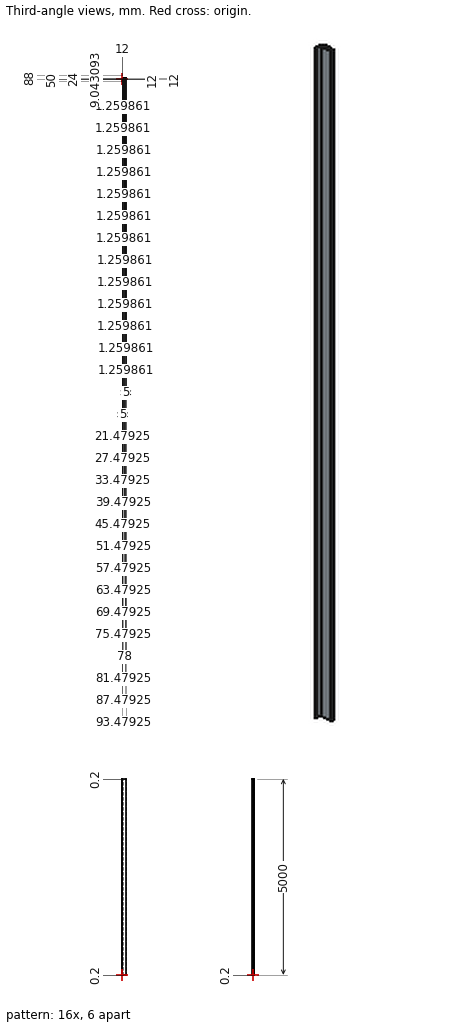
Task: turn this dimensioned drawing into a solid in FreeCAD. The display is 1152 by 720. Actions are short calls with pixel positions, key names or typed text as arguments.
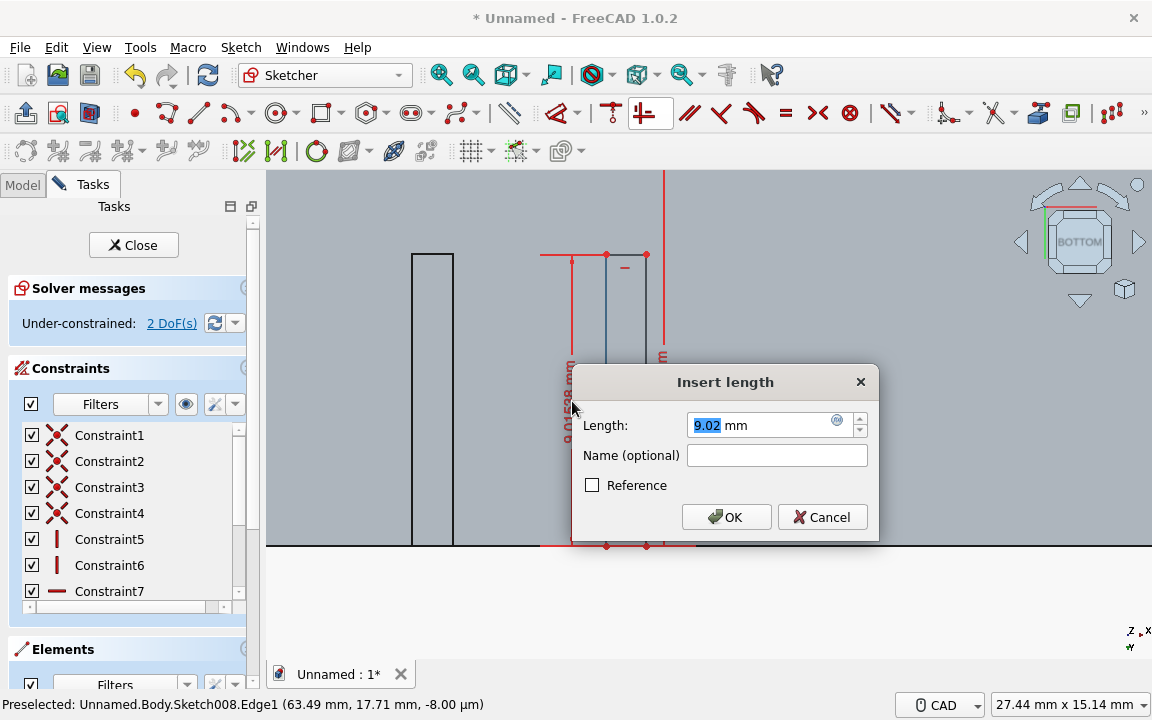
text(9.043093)
key(Return)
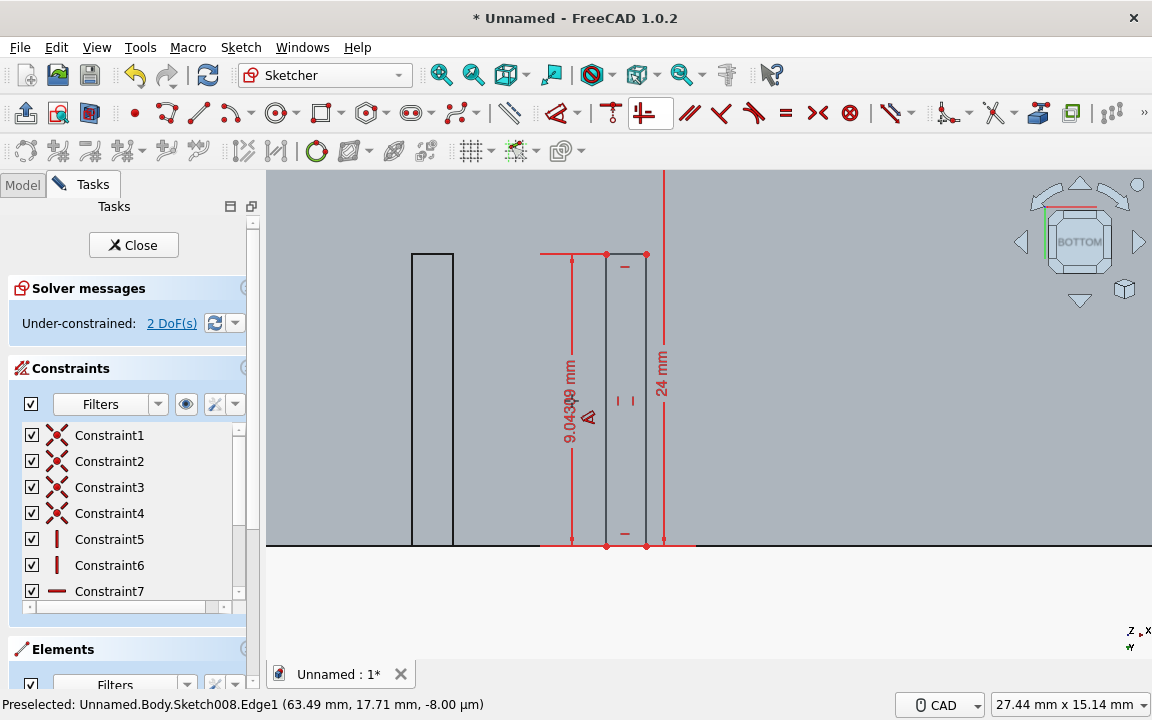
click(618, 546)
click(626, 580)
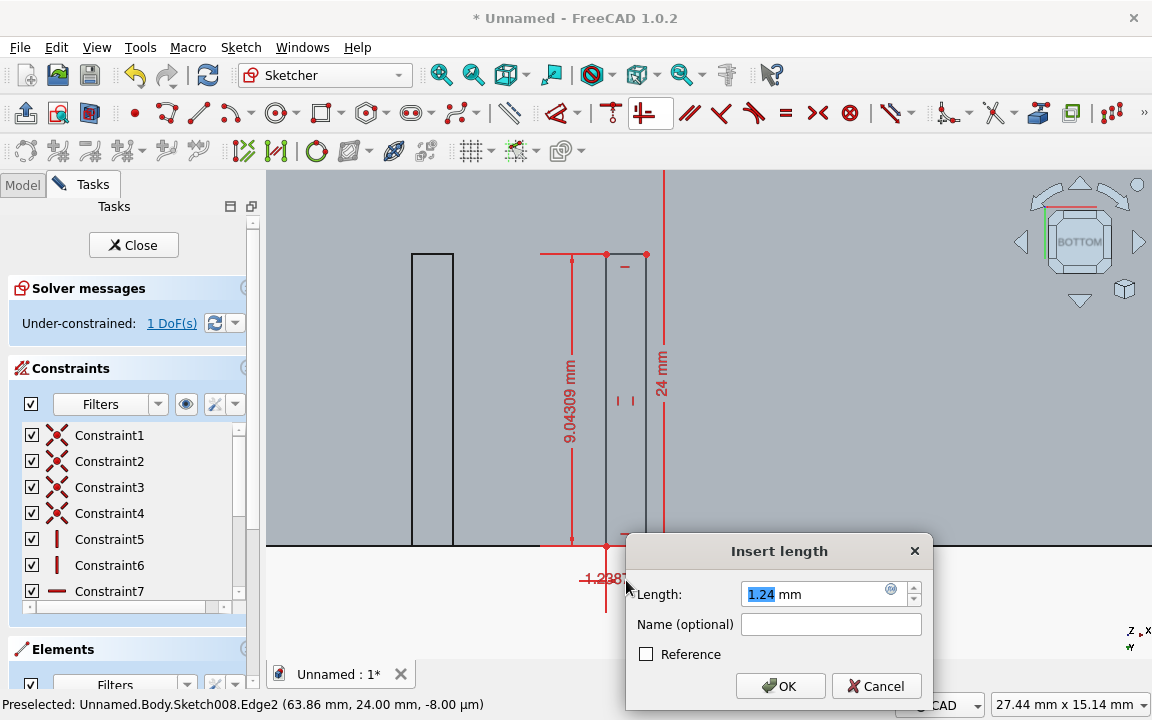
text(1.259861)
key(Return)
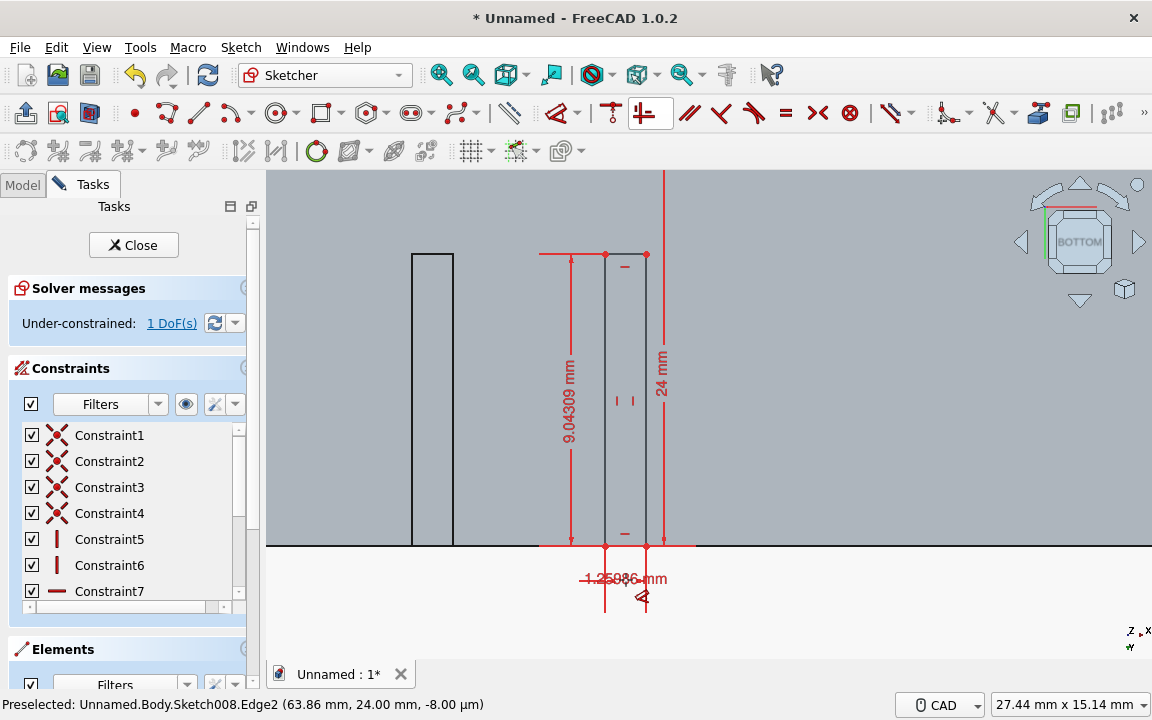
click(605, 254)
click(450, 288)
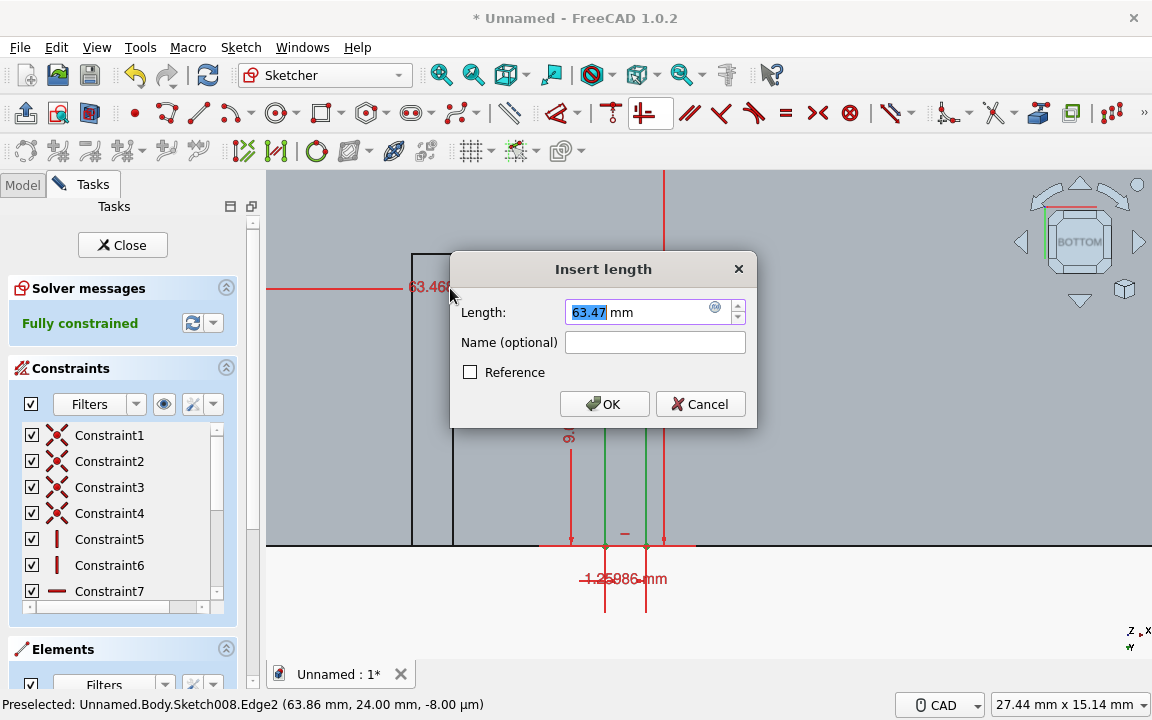
text(63.47925)
key(Return)
key(Escape)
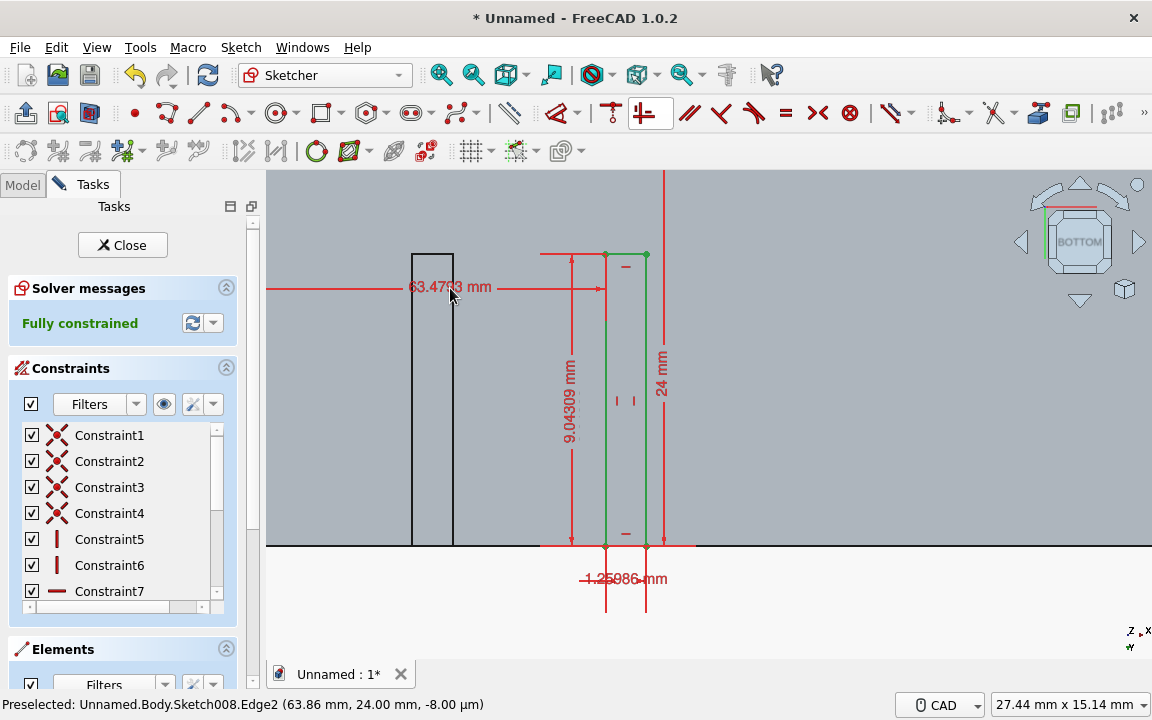
click(123, 245)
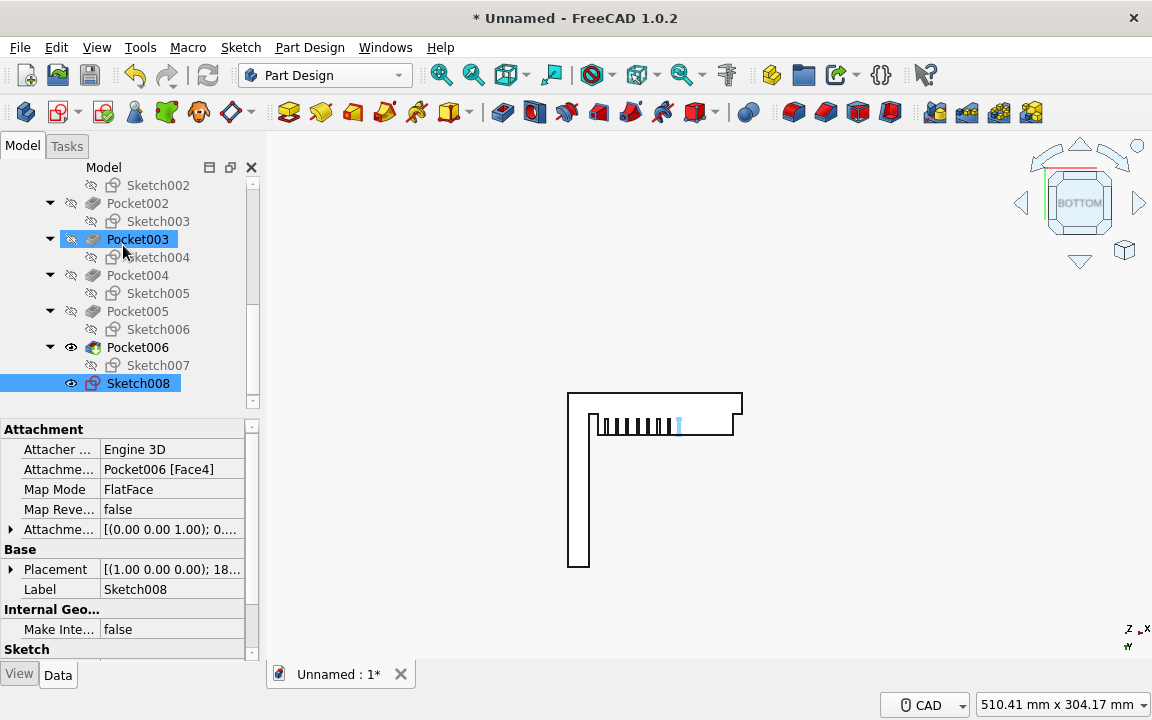
click(504, 112)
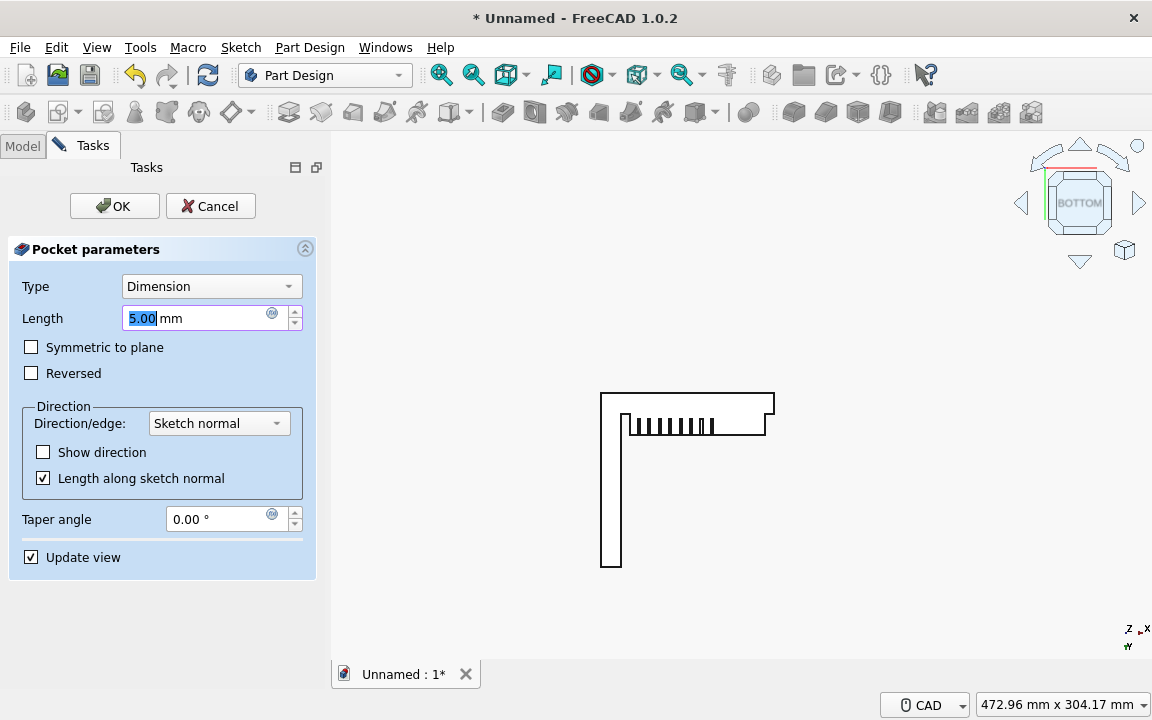
text(0.2)
key(Tab)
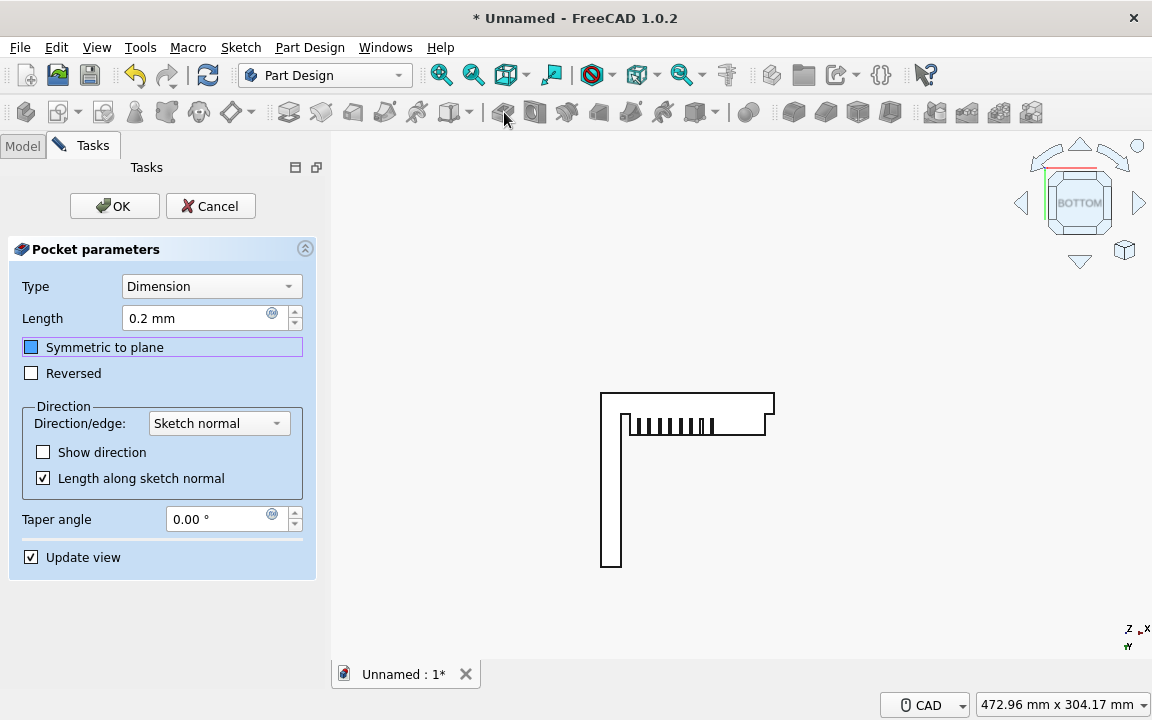
click(115, 206)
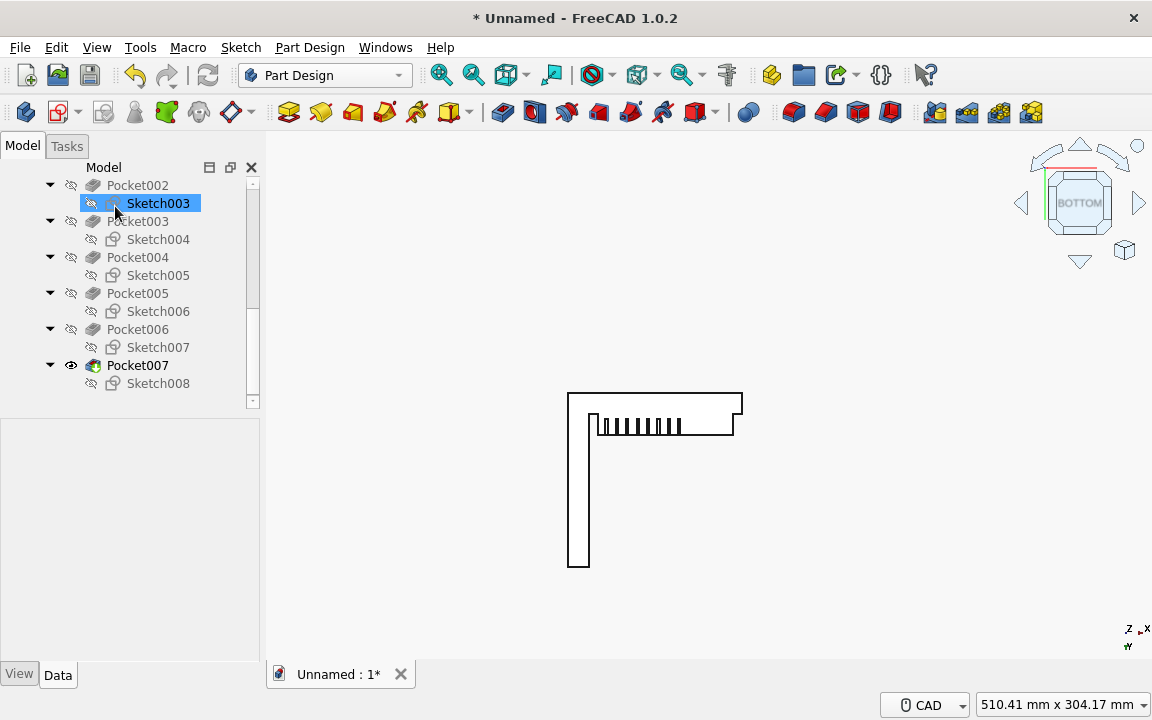
click(442, 76)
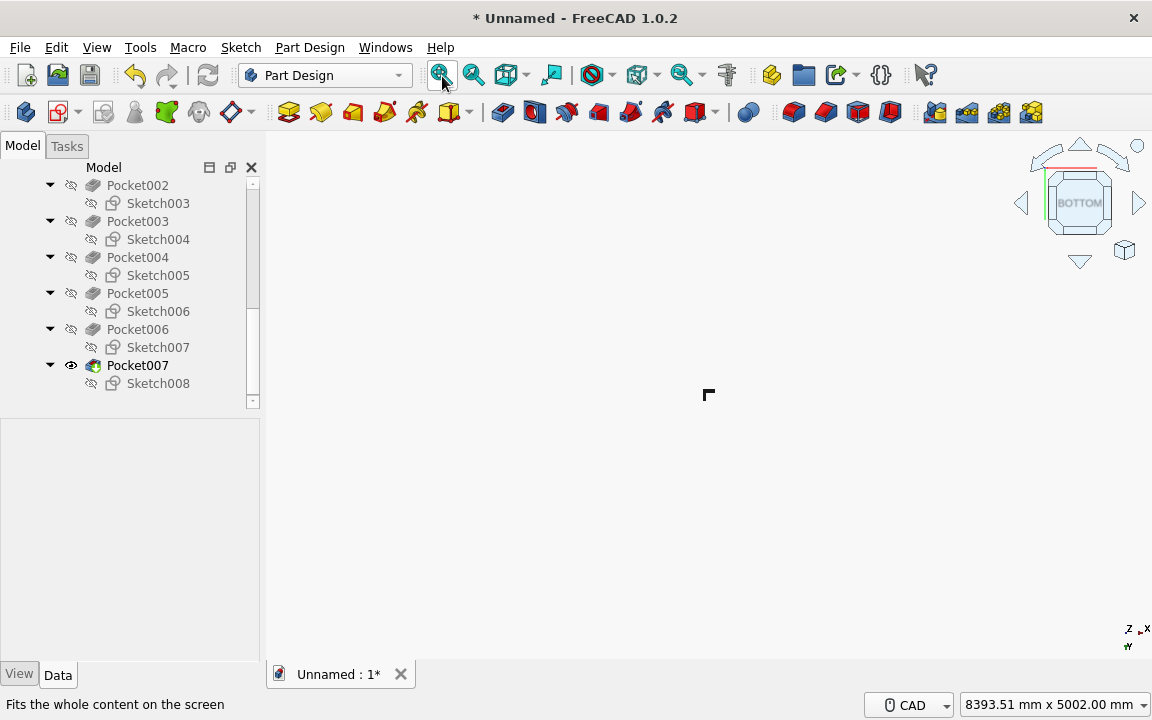
scroll(712, 389, up, 14)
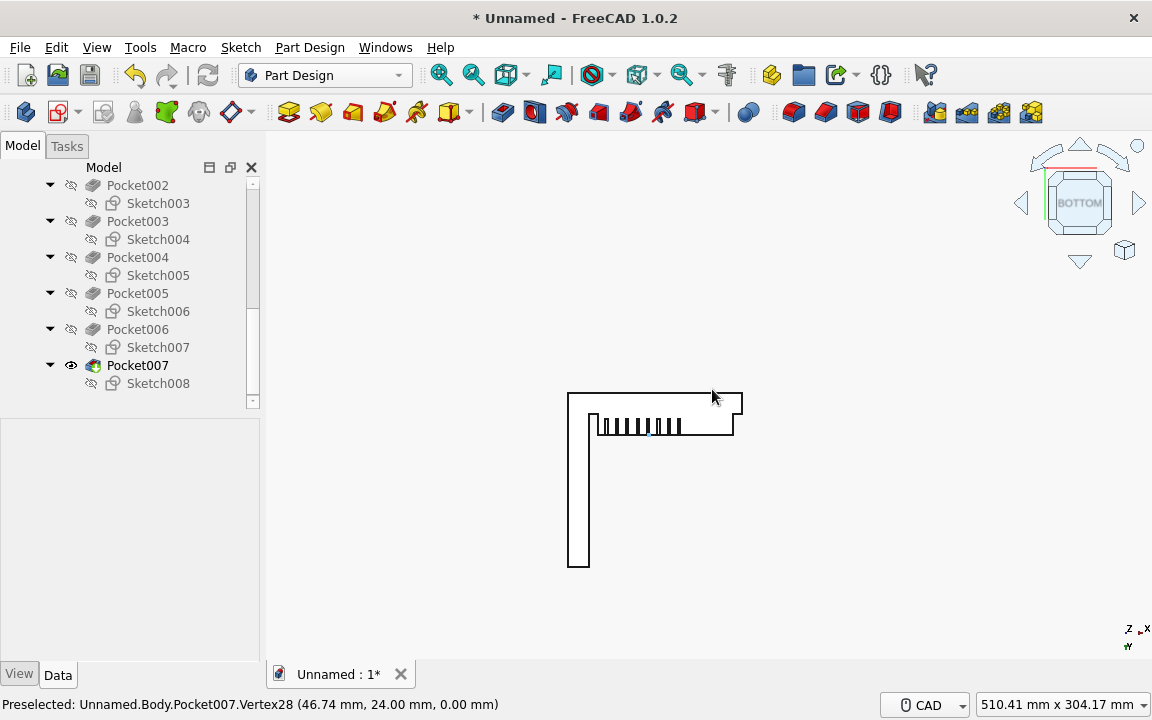
click(704, 405)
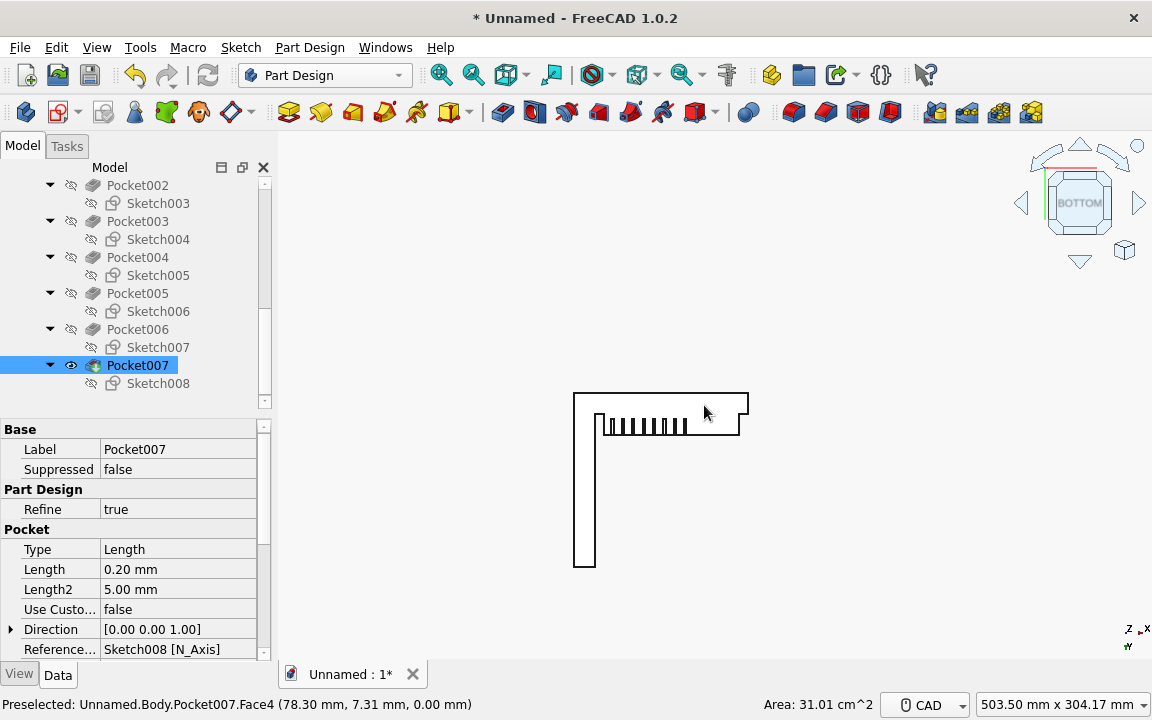
click(58, 112)